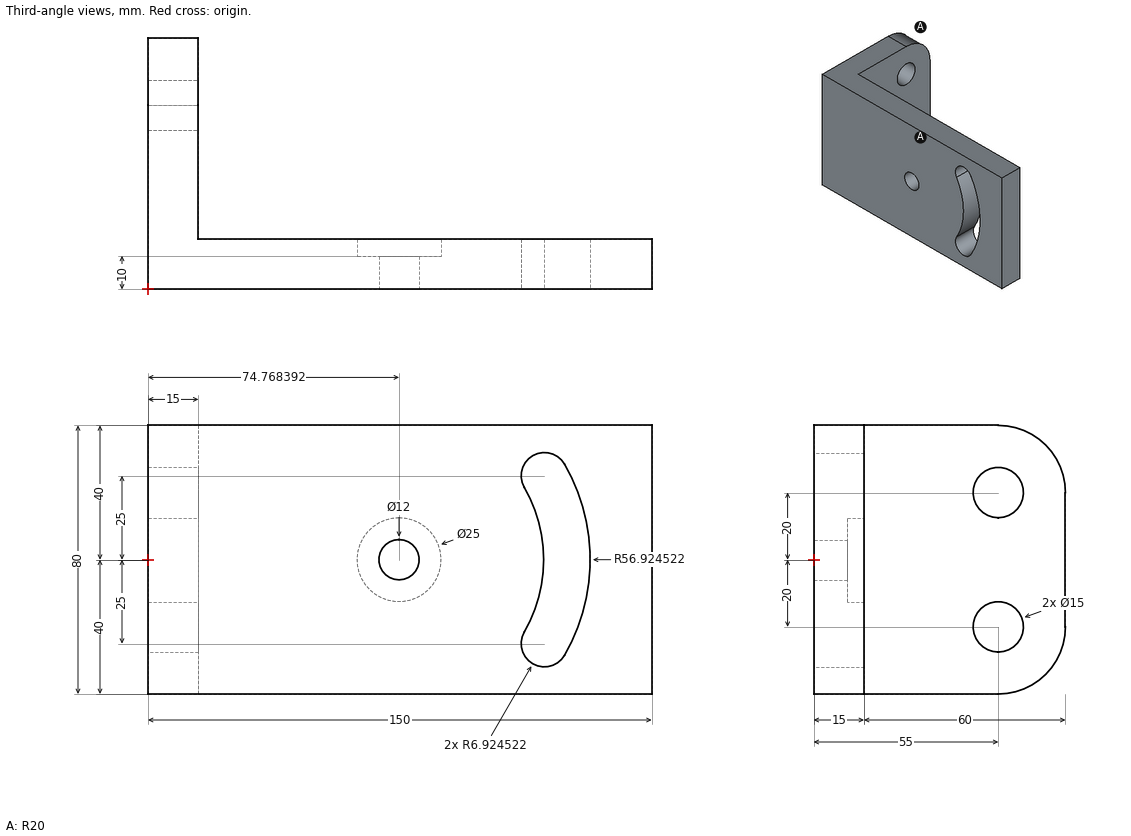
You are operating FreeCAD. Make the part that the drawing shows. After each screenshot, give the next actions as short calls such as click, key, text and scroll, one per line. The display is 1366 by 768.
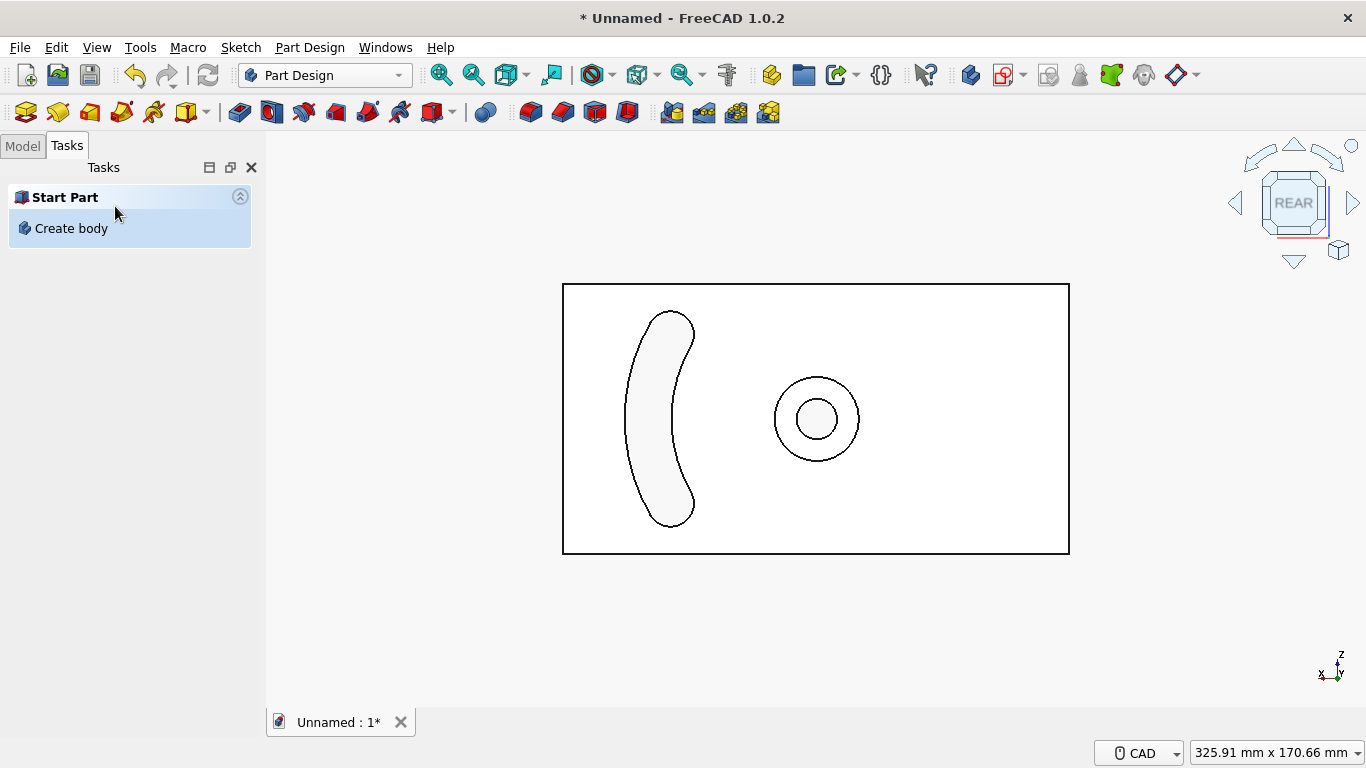
click(961, 418)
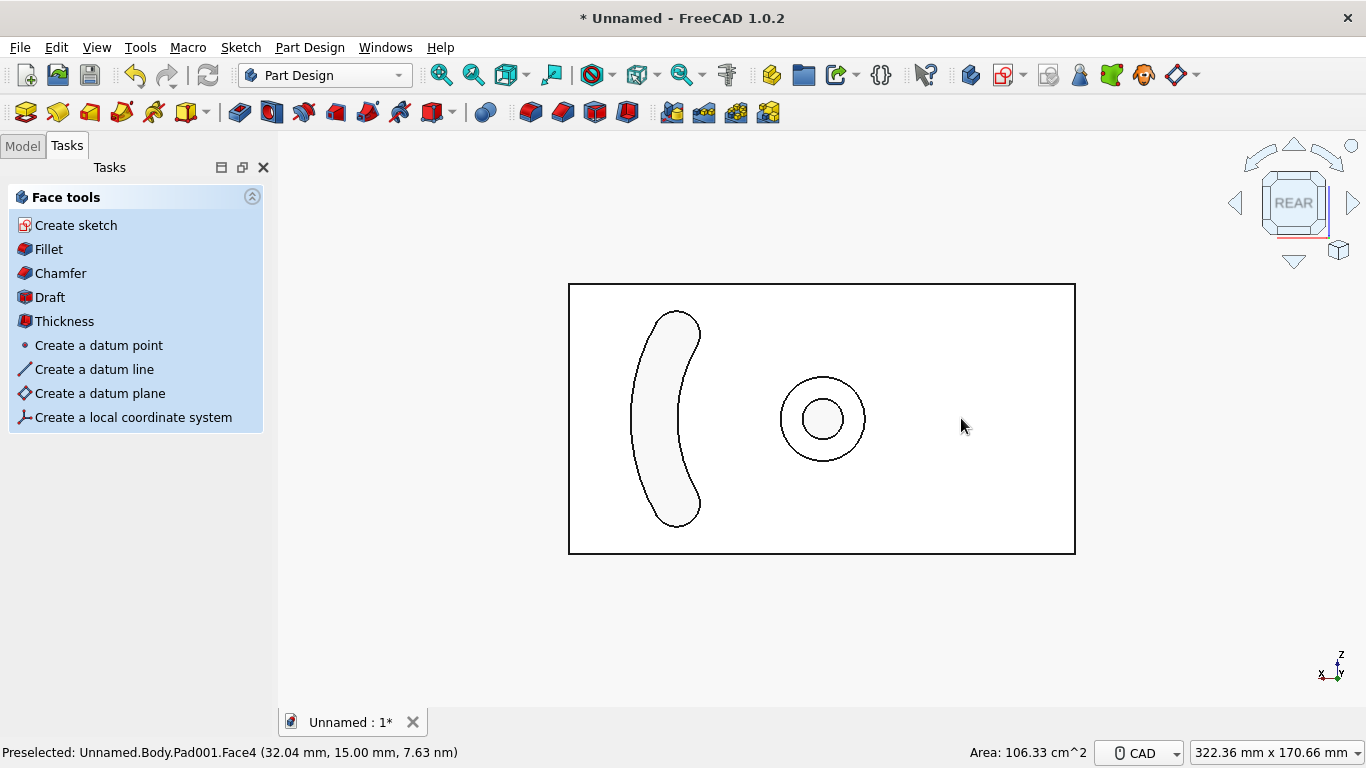
click(1004, 76)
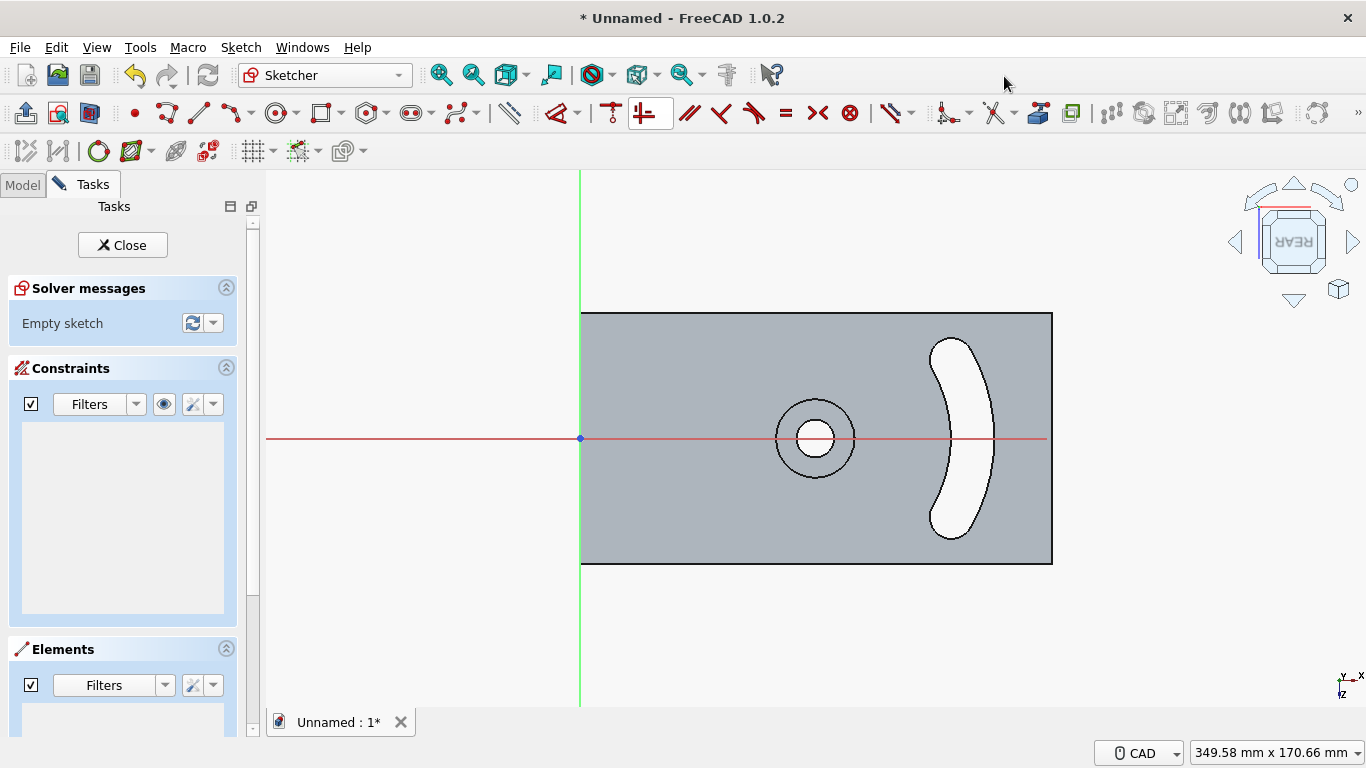
key(g)
key(r)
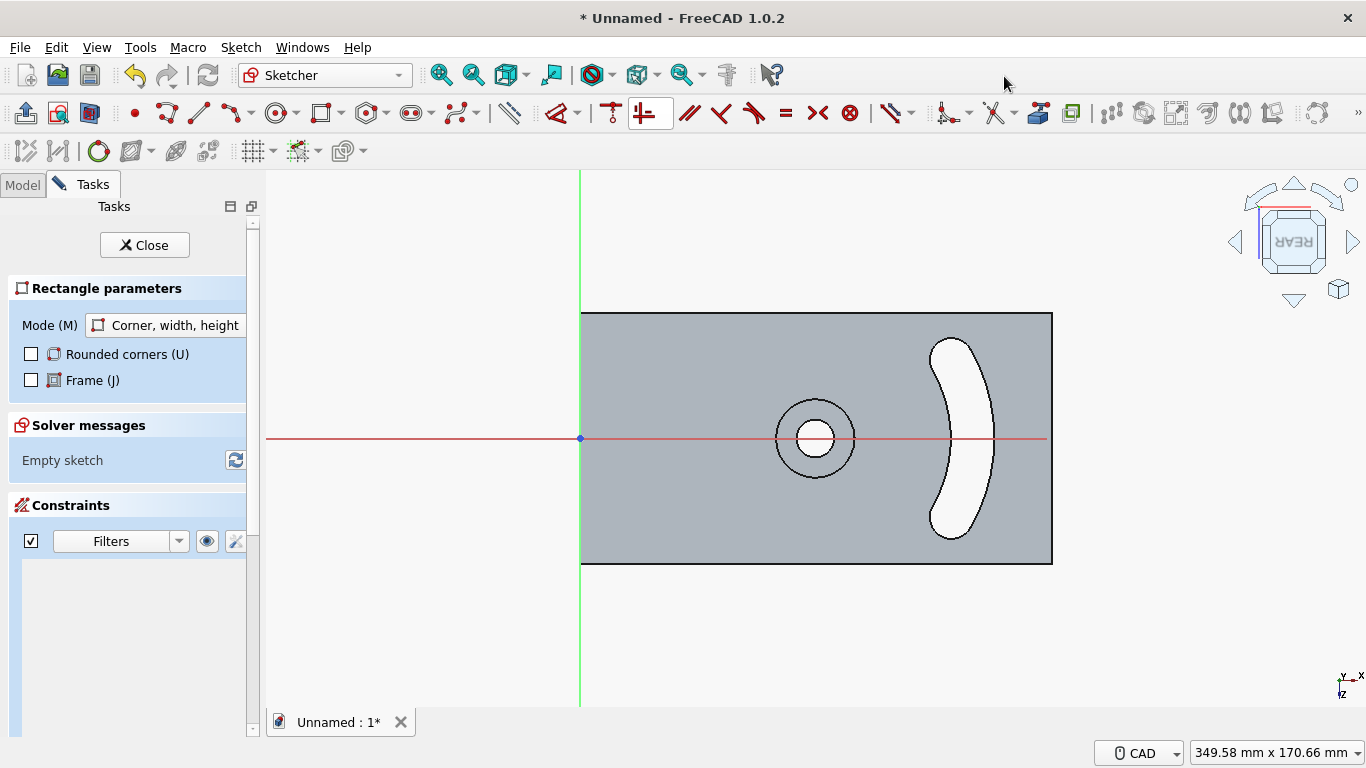
click(580, 313)
click(627, 564)
key(Escape)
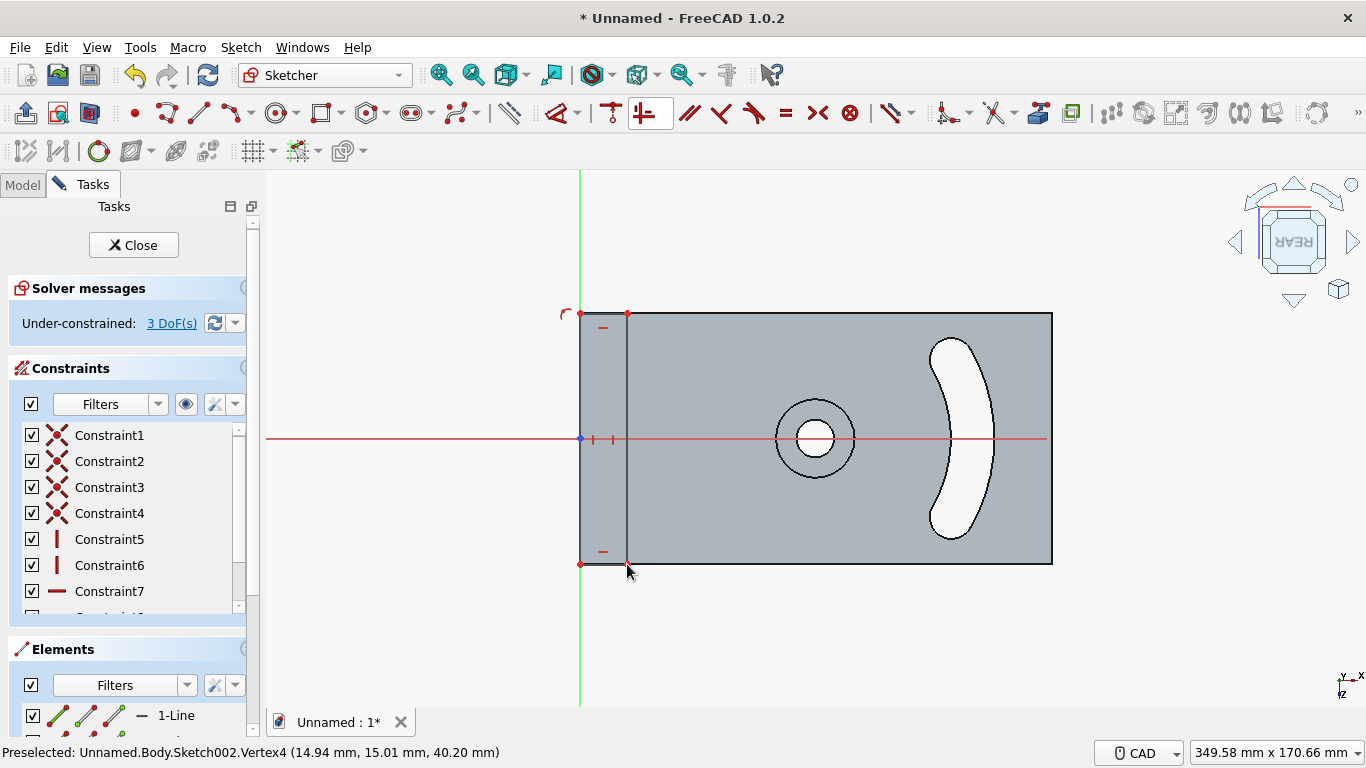
click(556, 114)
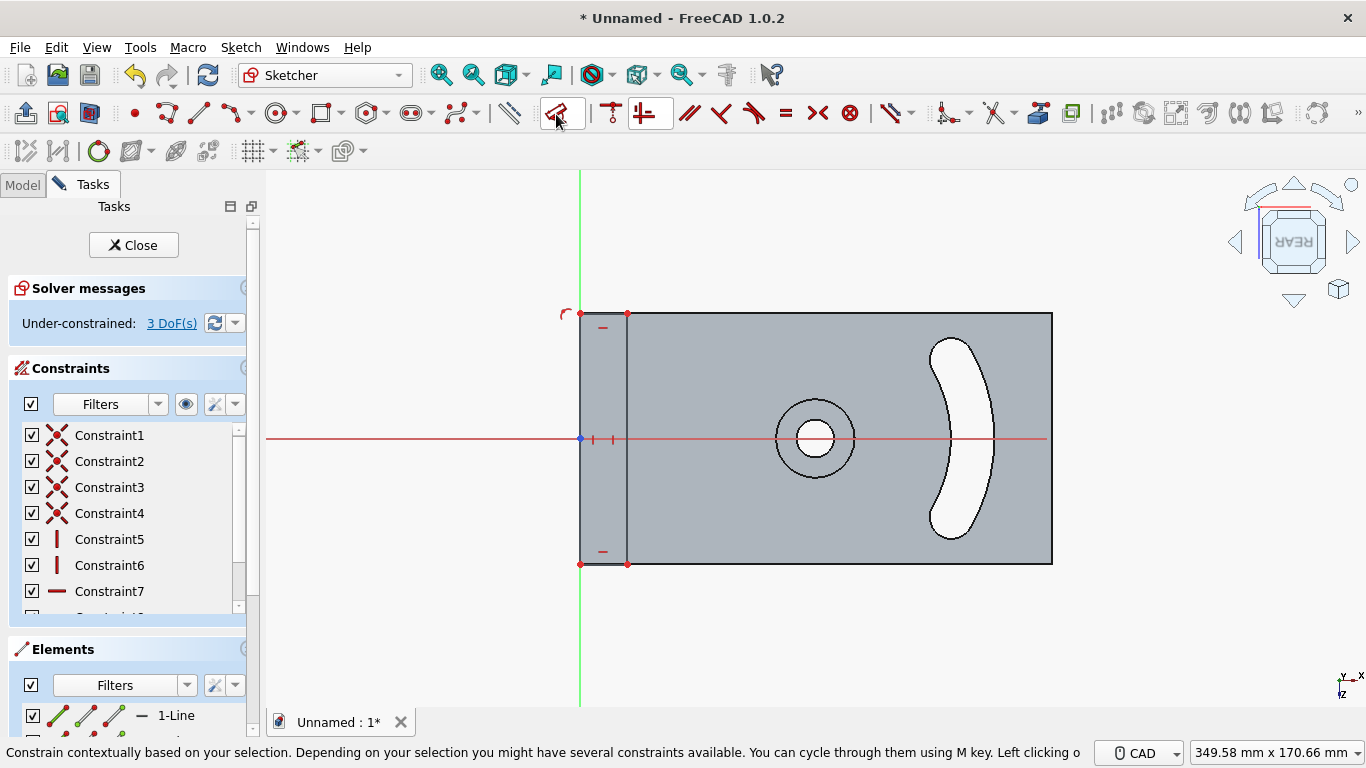
click(580, 389)
click(546, 382)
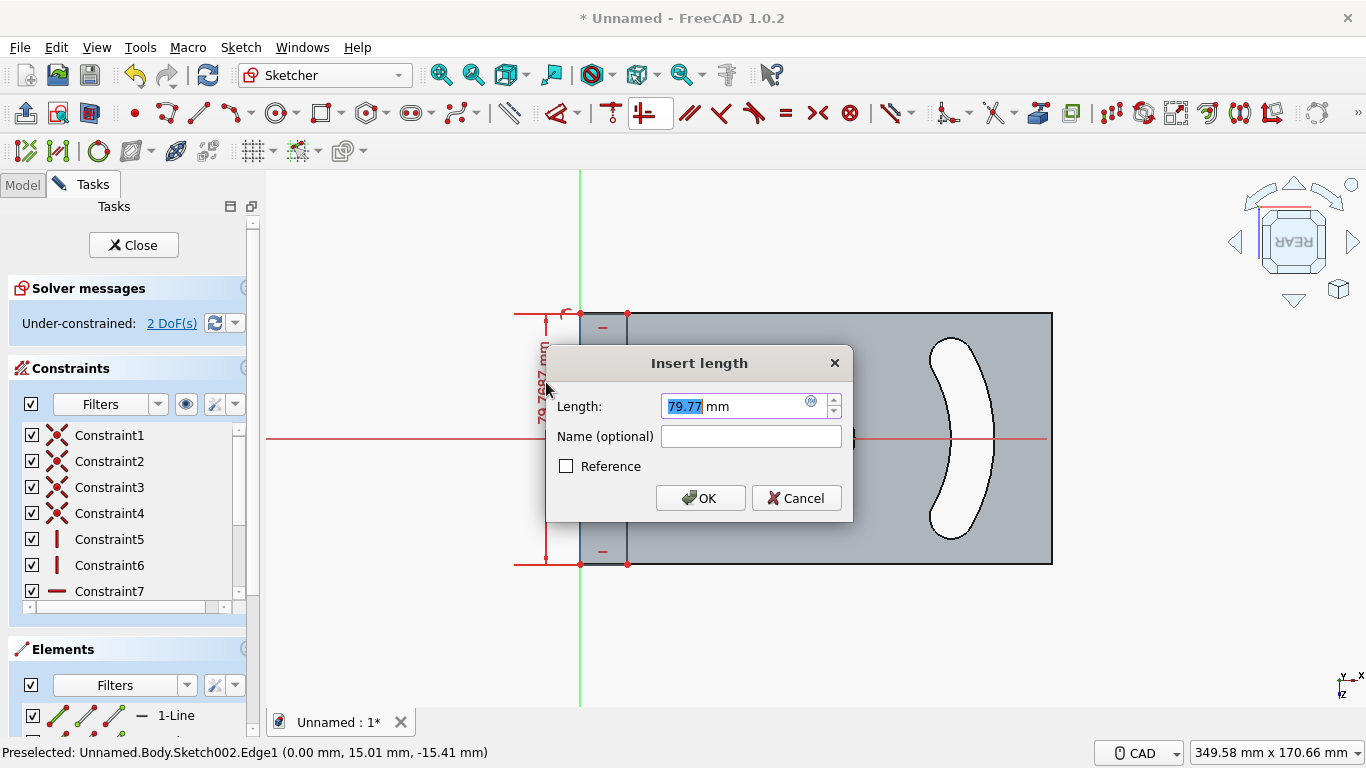
text(80)
key(Return)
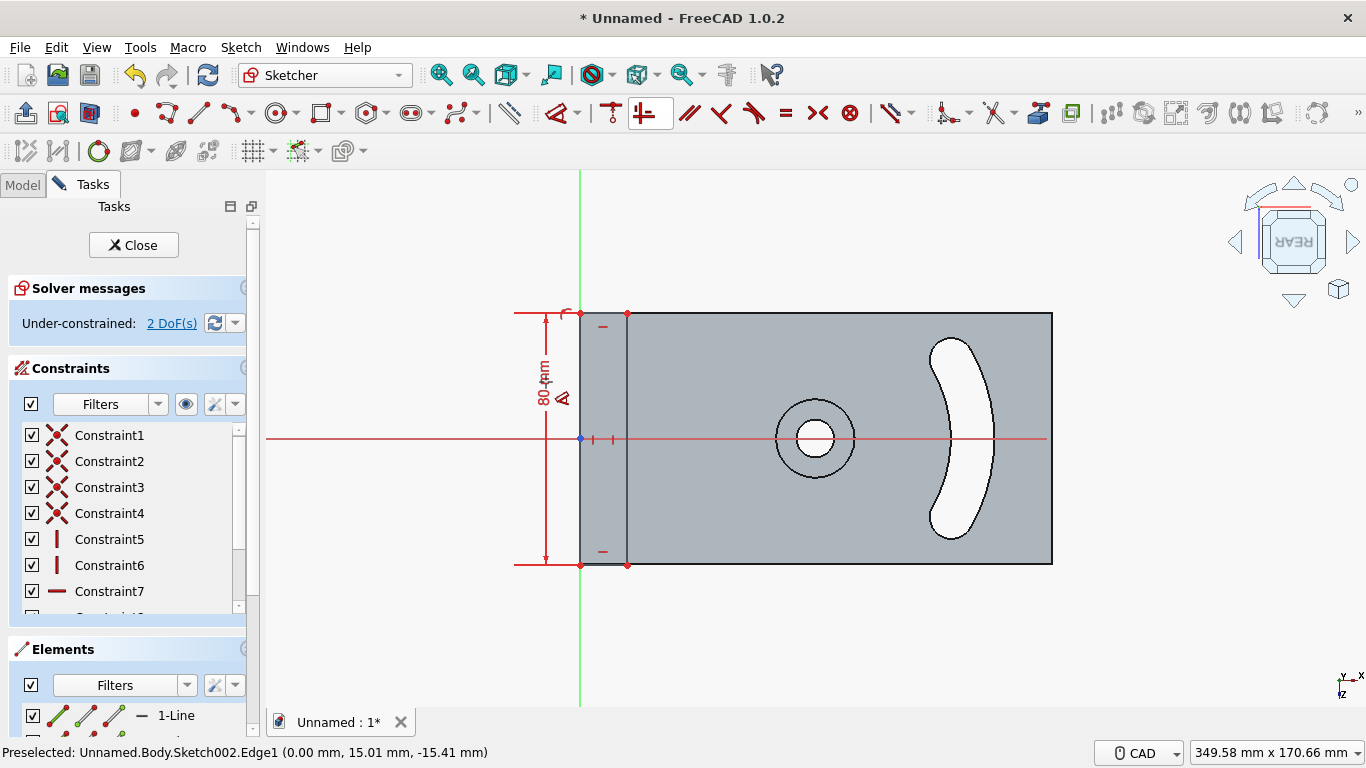
click(594, 565)
click(604, 599)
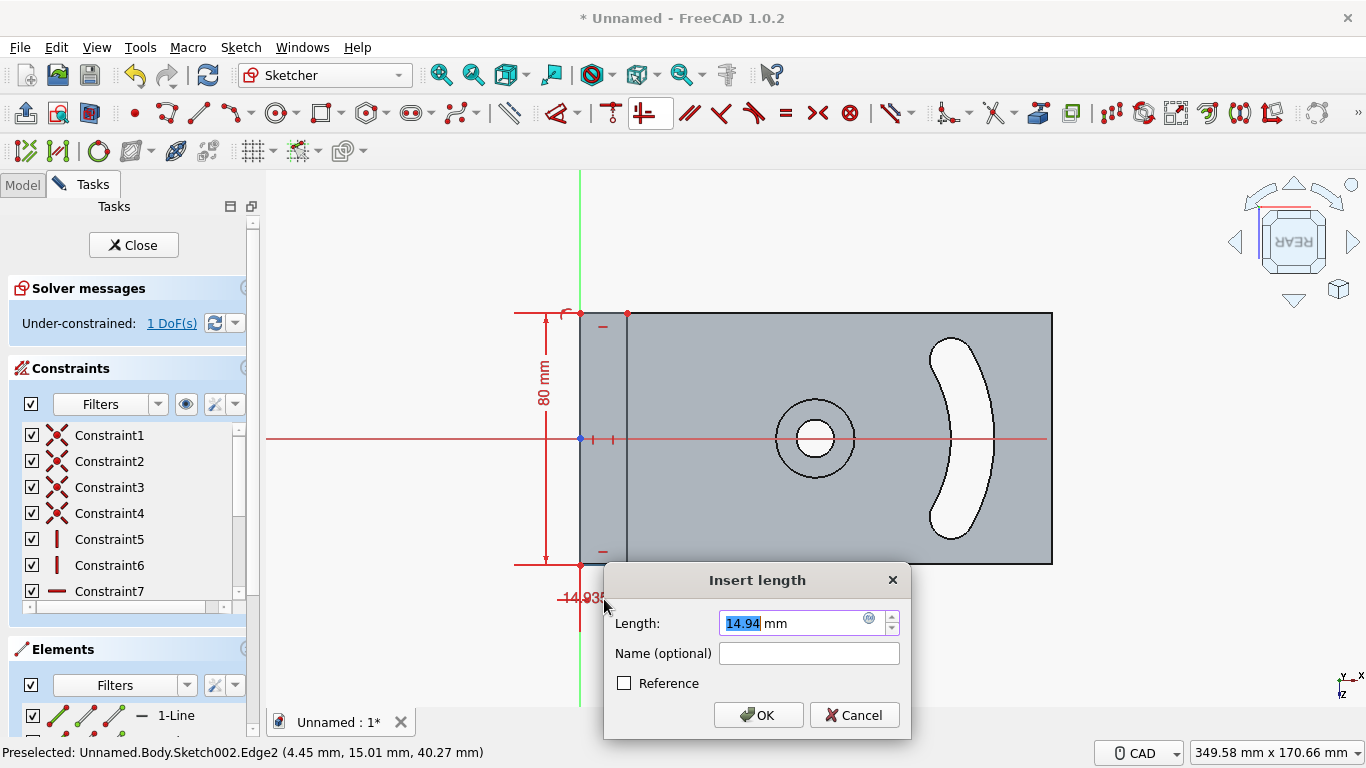
text(15)
key(Return)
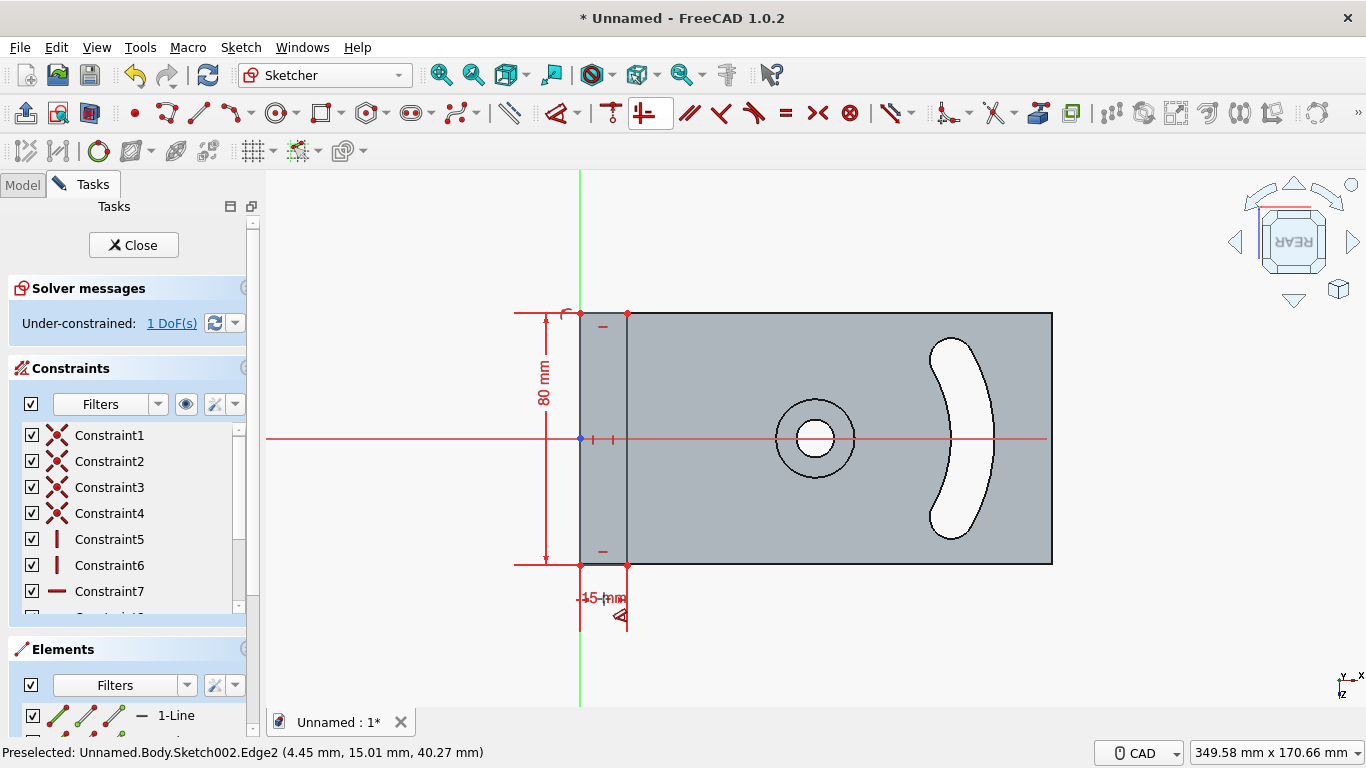
click(580, 313)
click(546, 347)